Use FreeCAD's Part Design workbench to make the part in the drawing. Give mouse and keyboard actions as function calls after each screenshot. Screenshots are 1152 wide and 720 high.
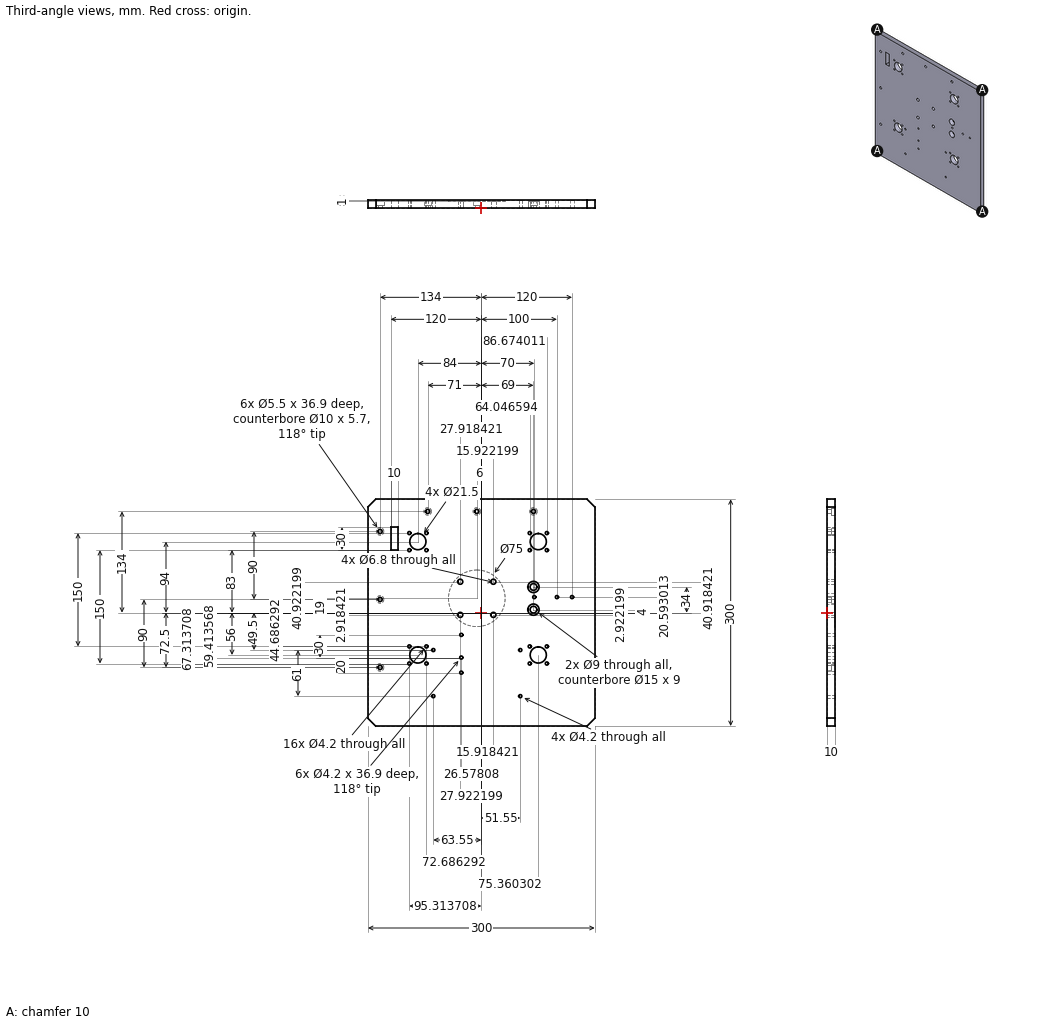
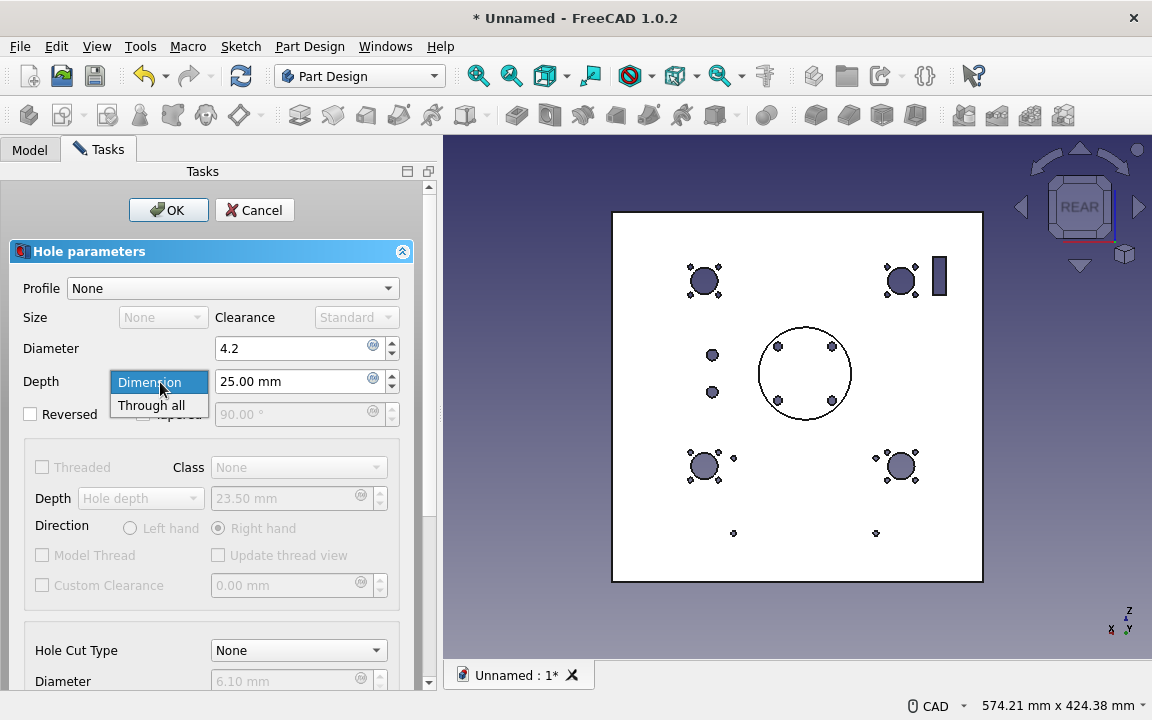
click(158, 406)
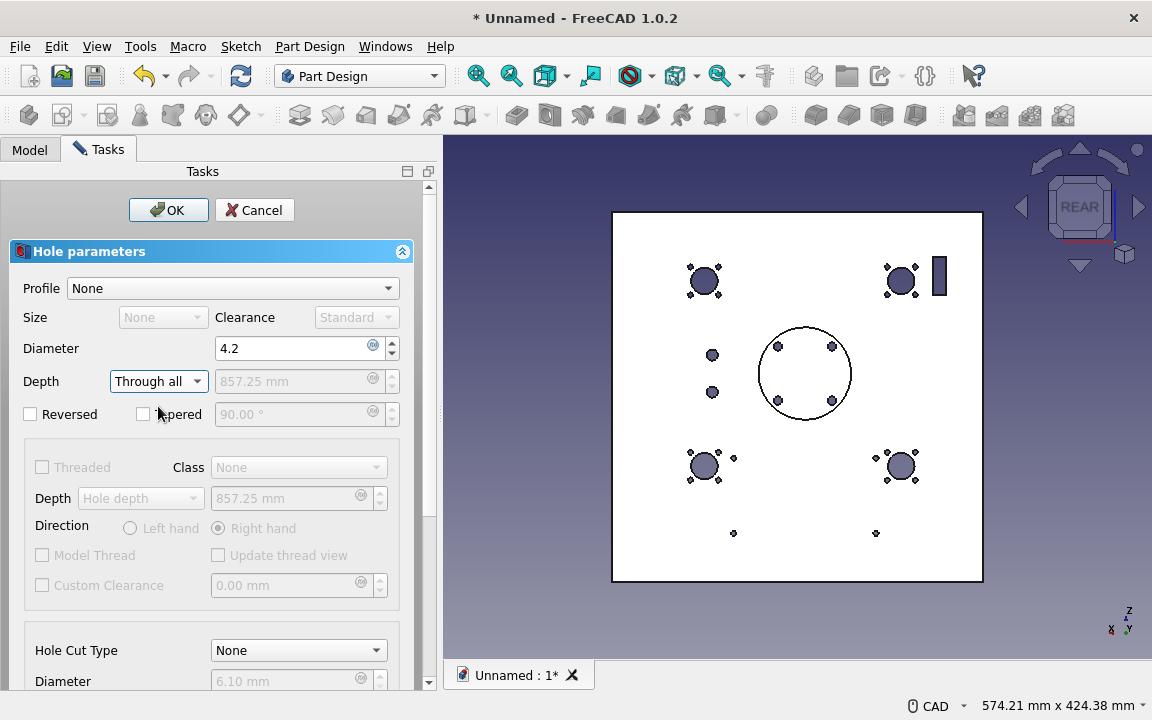
click(169, 210)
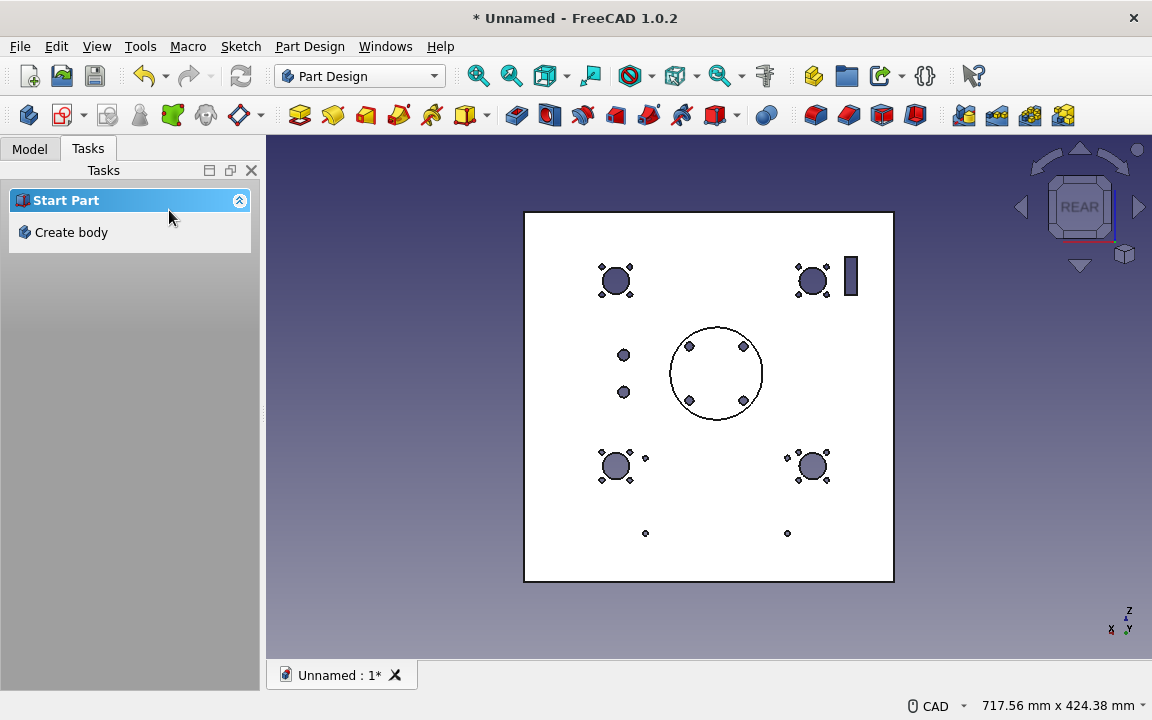
scroll(524, 211, up, 6)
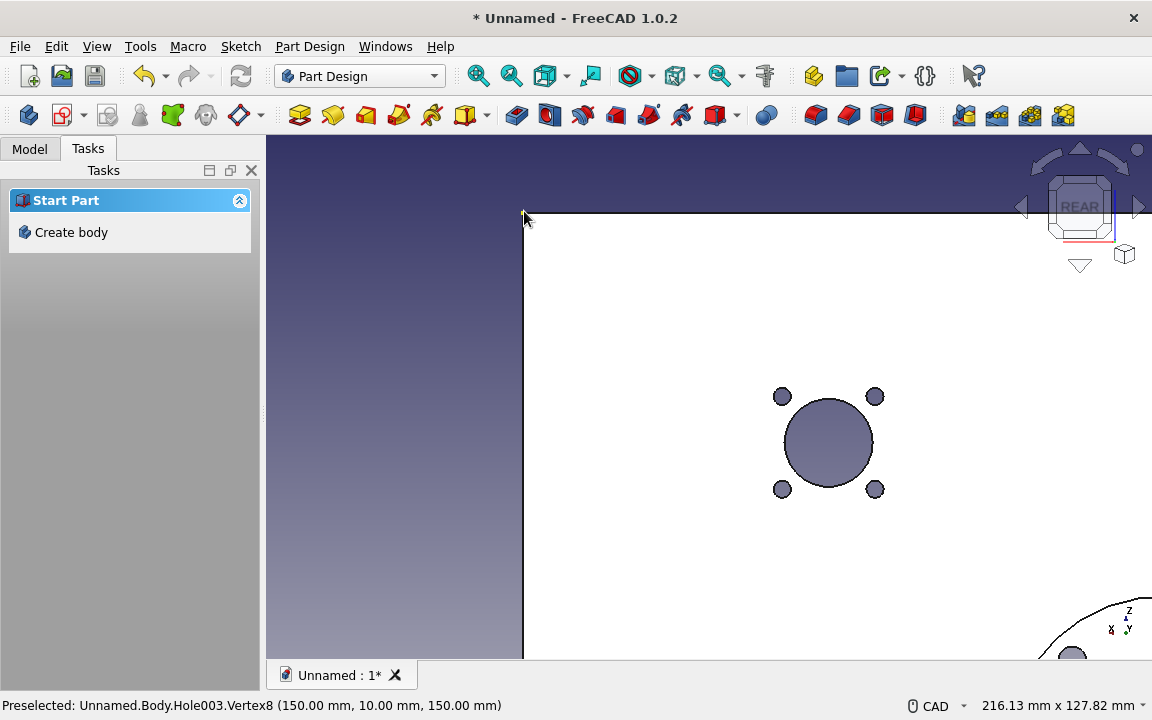
click(479, 76)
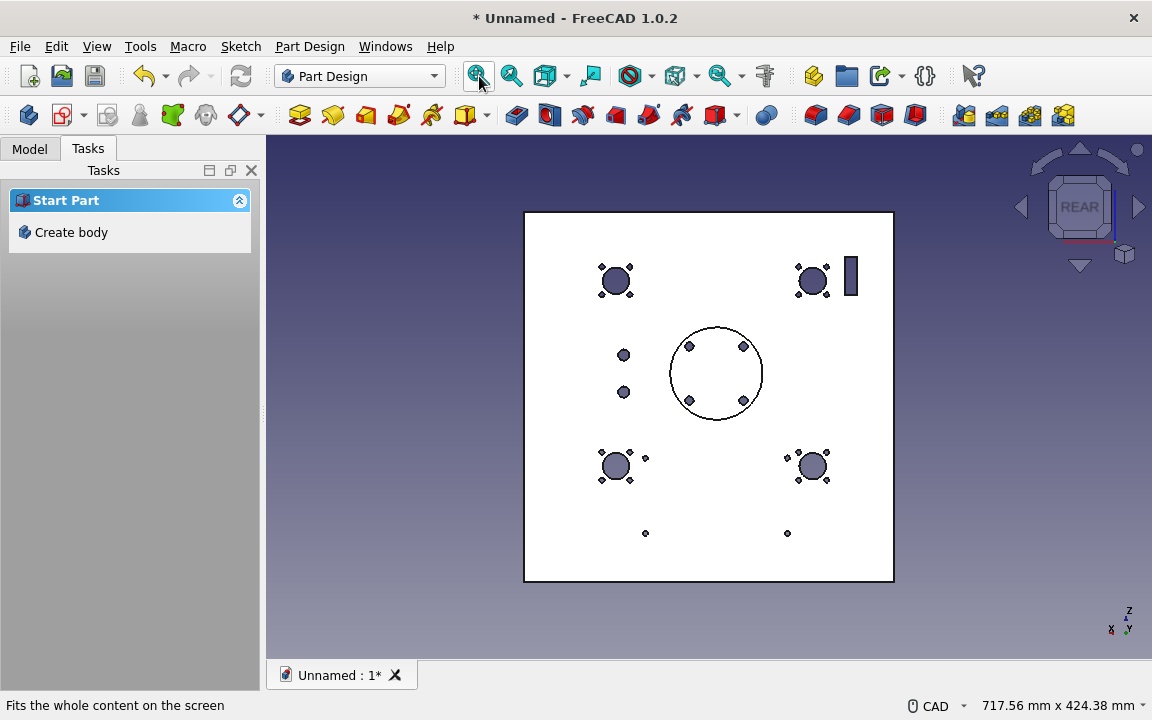
key(0)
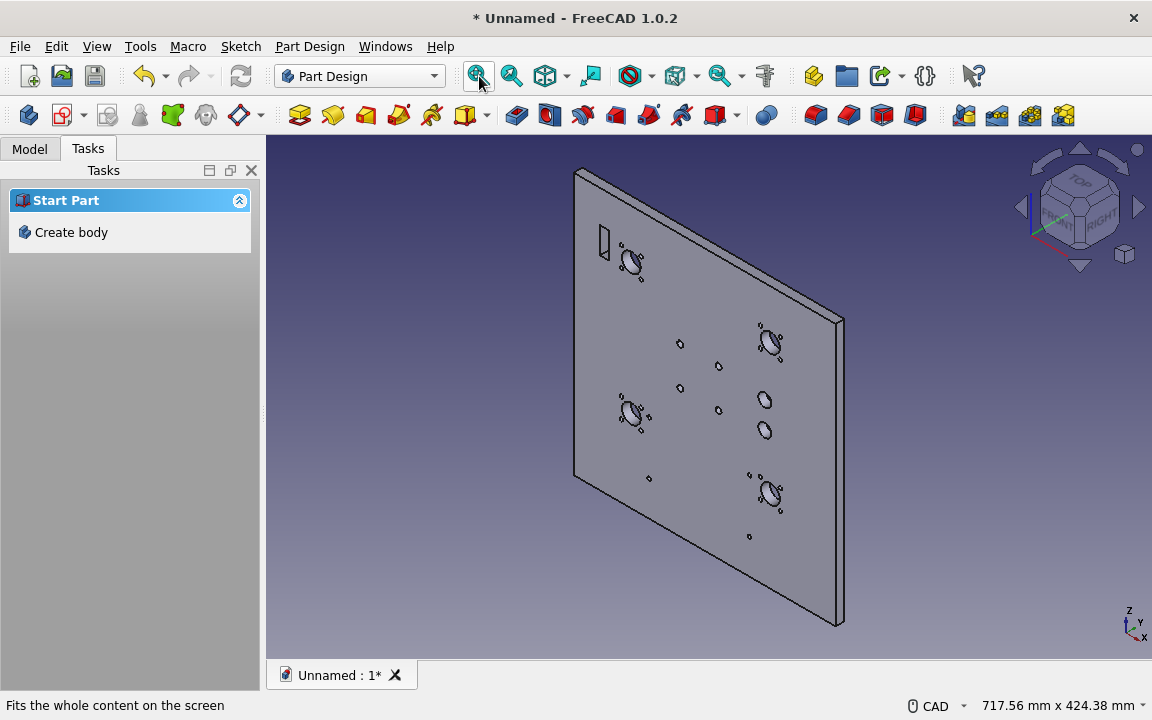
click(842, 319)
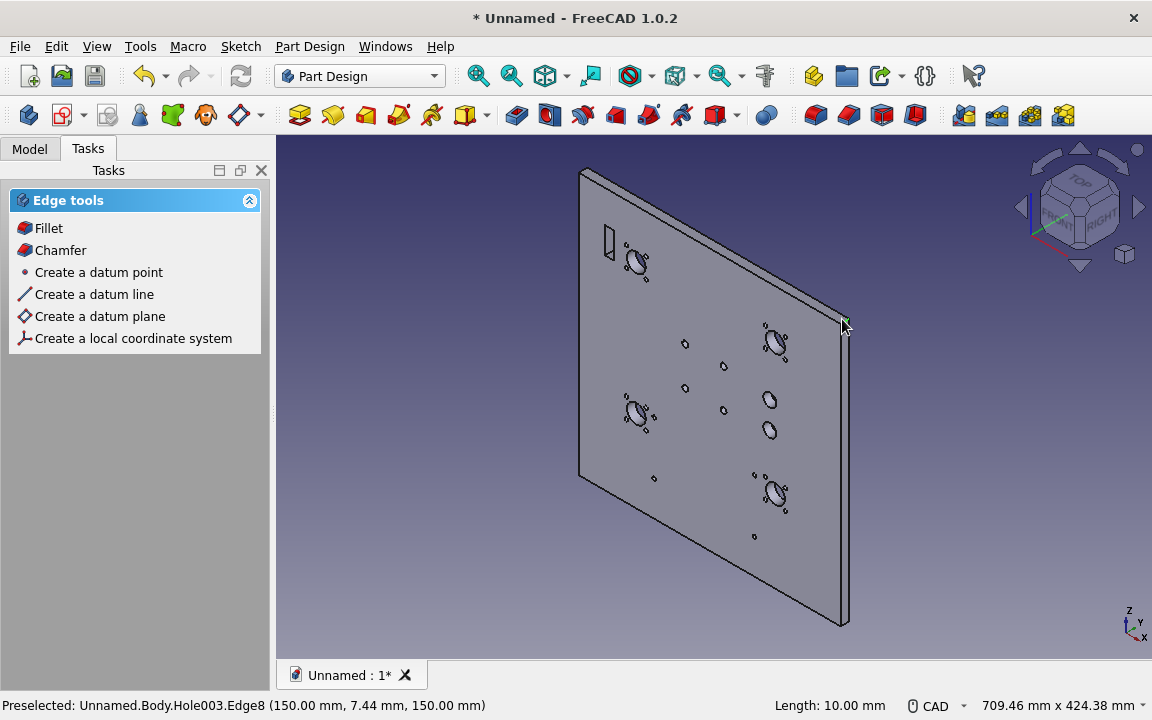
scroll(583, 169, up, 6)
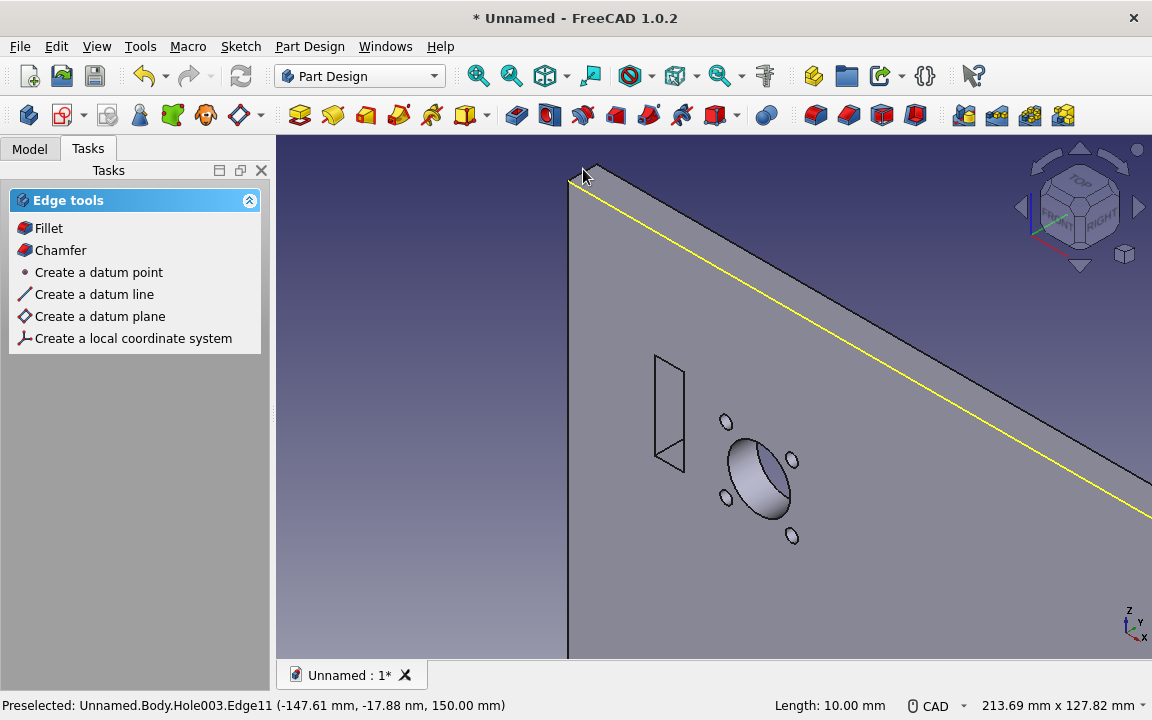
click(479, 76)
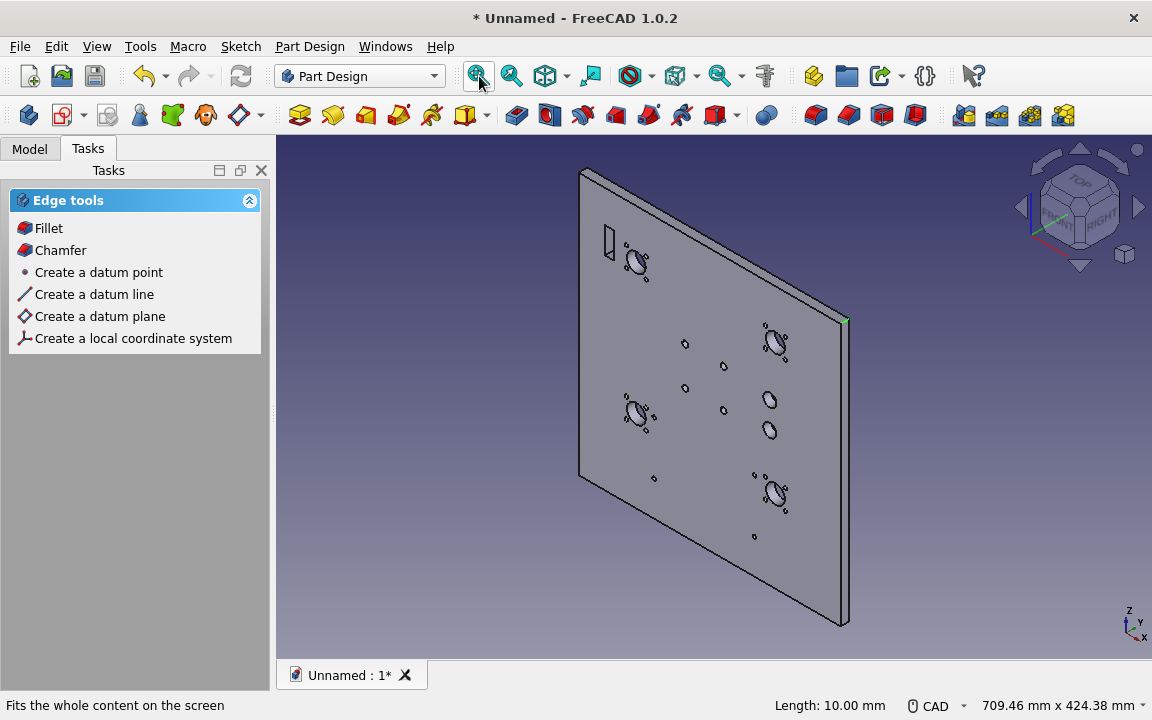
key(2)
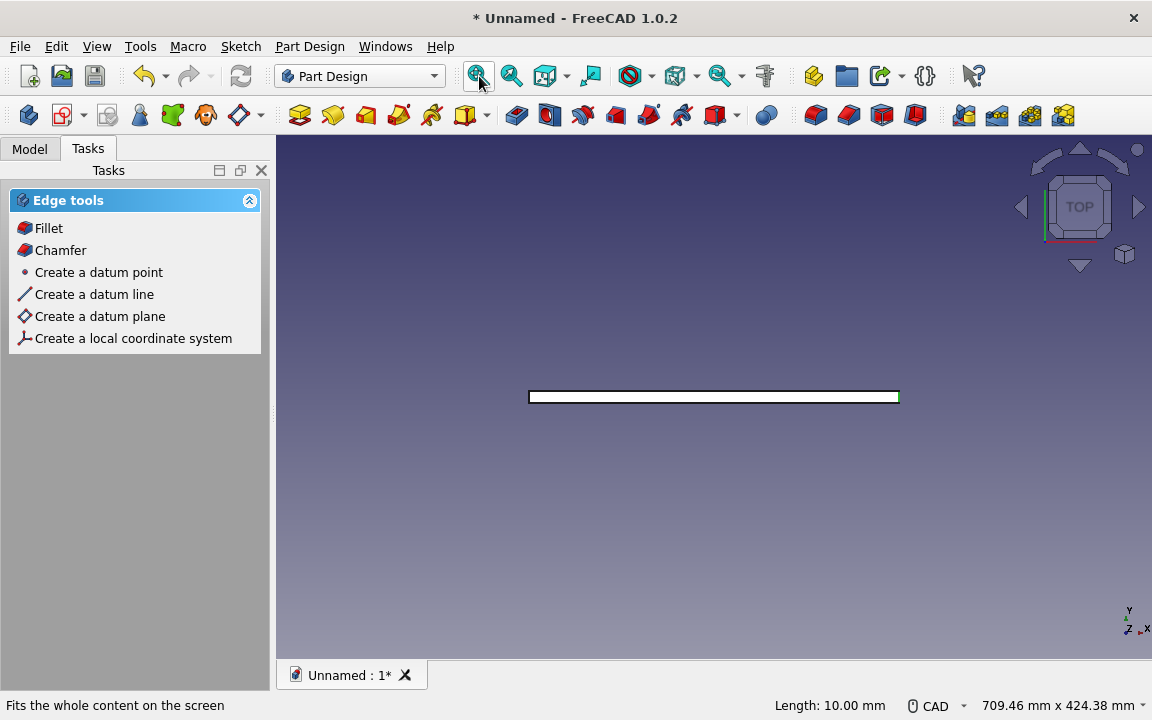
click(479, 76)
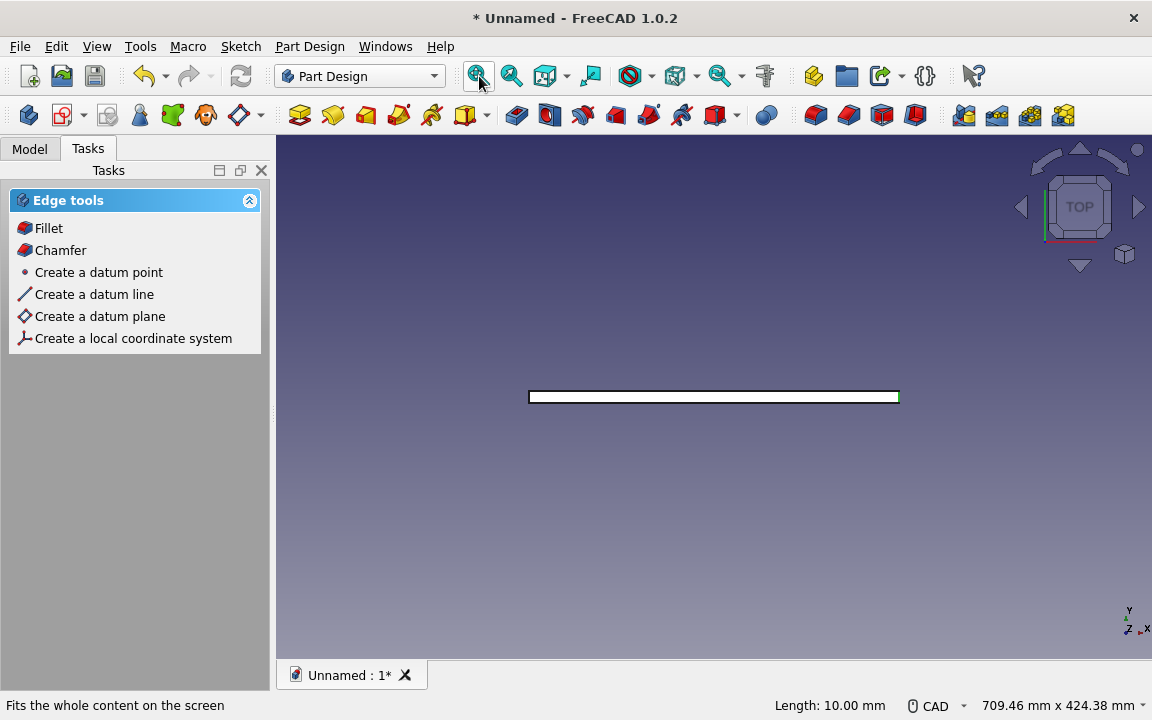
click(529, 396, ctrl)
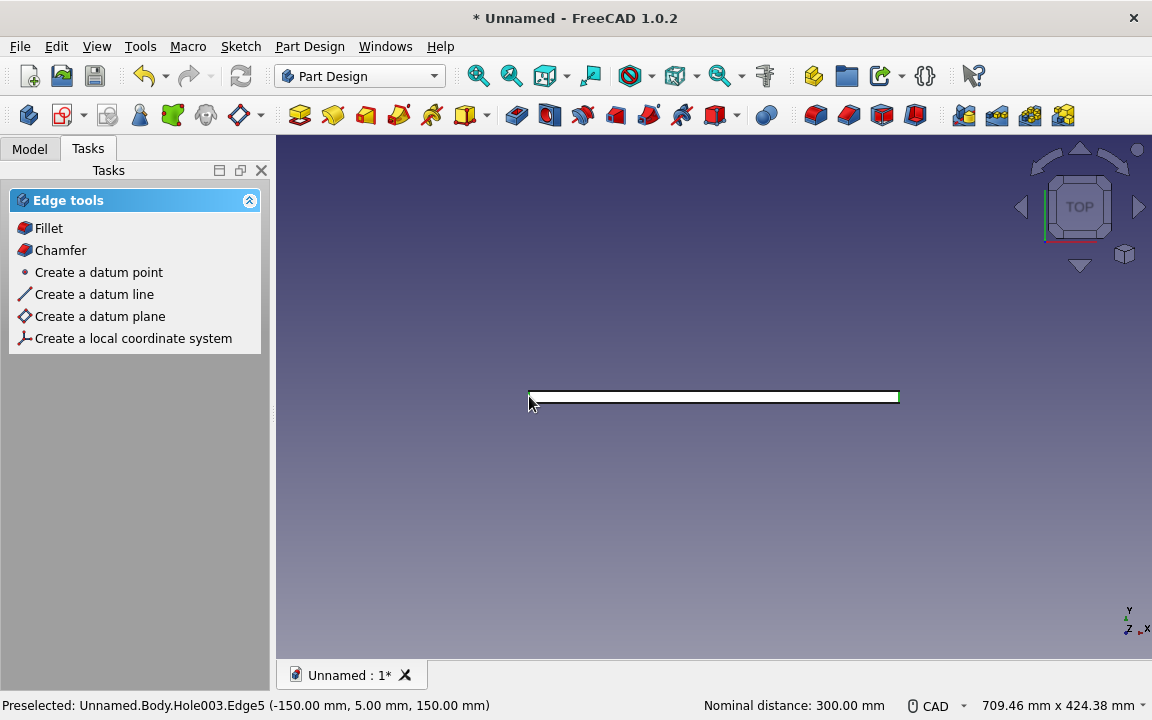
scroll(529, 396, up, 6)